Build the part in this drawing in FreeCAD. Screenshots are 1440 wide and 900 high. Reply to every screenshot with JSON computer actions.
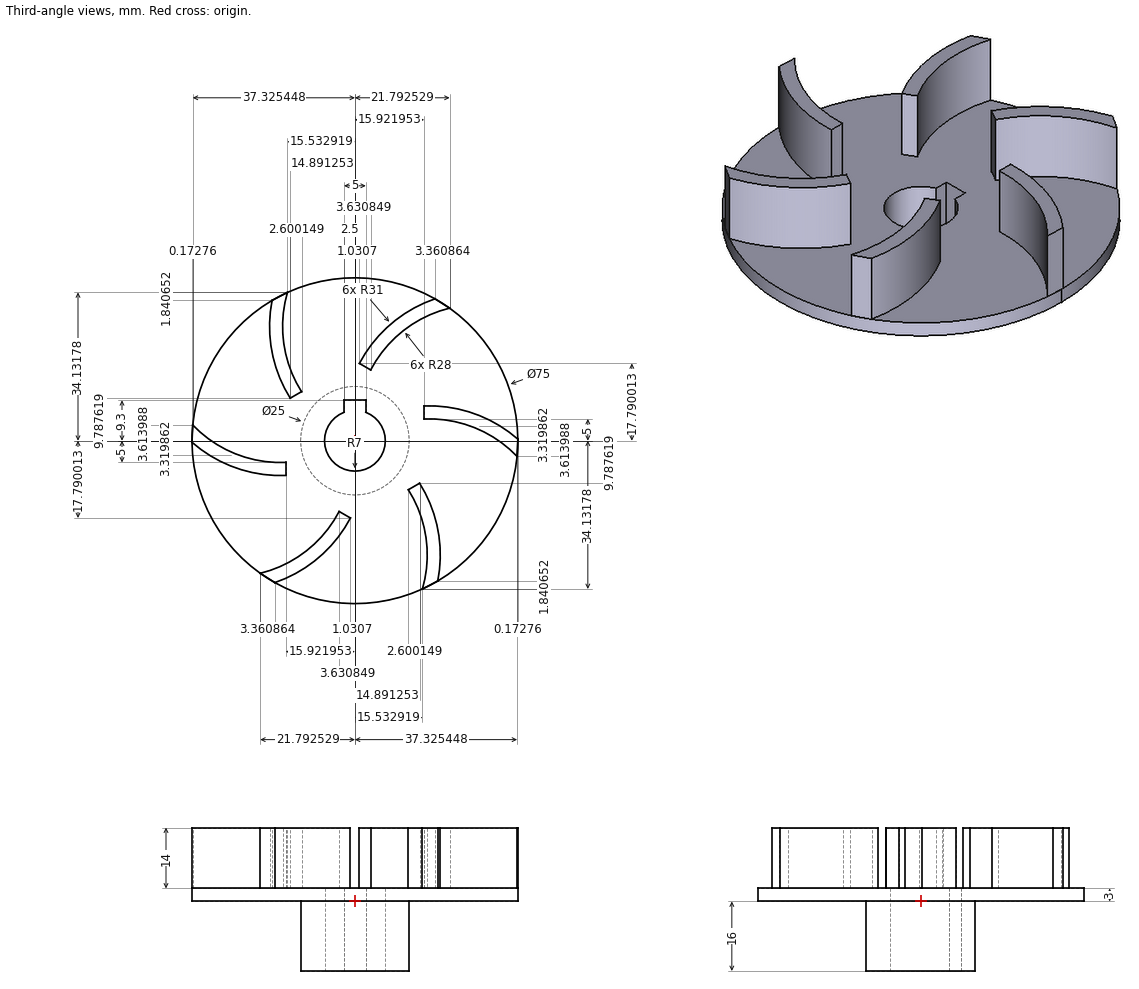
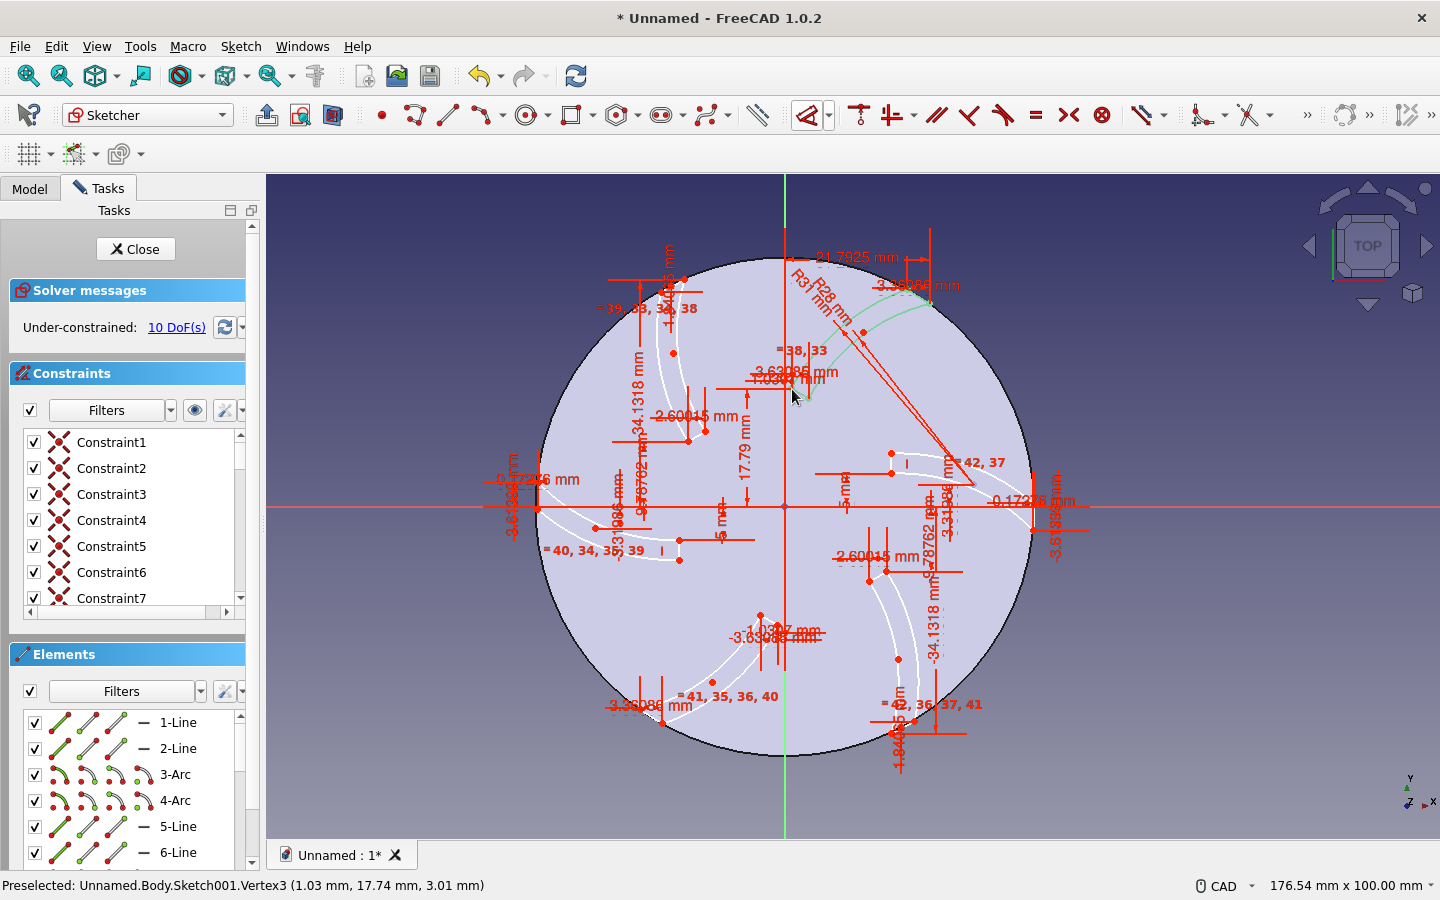
{"action": "left_click", "coordinate": [685, 280]}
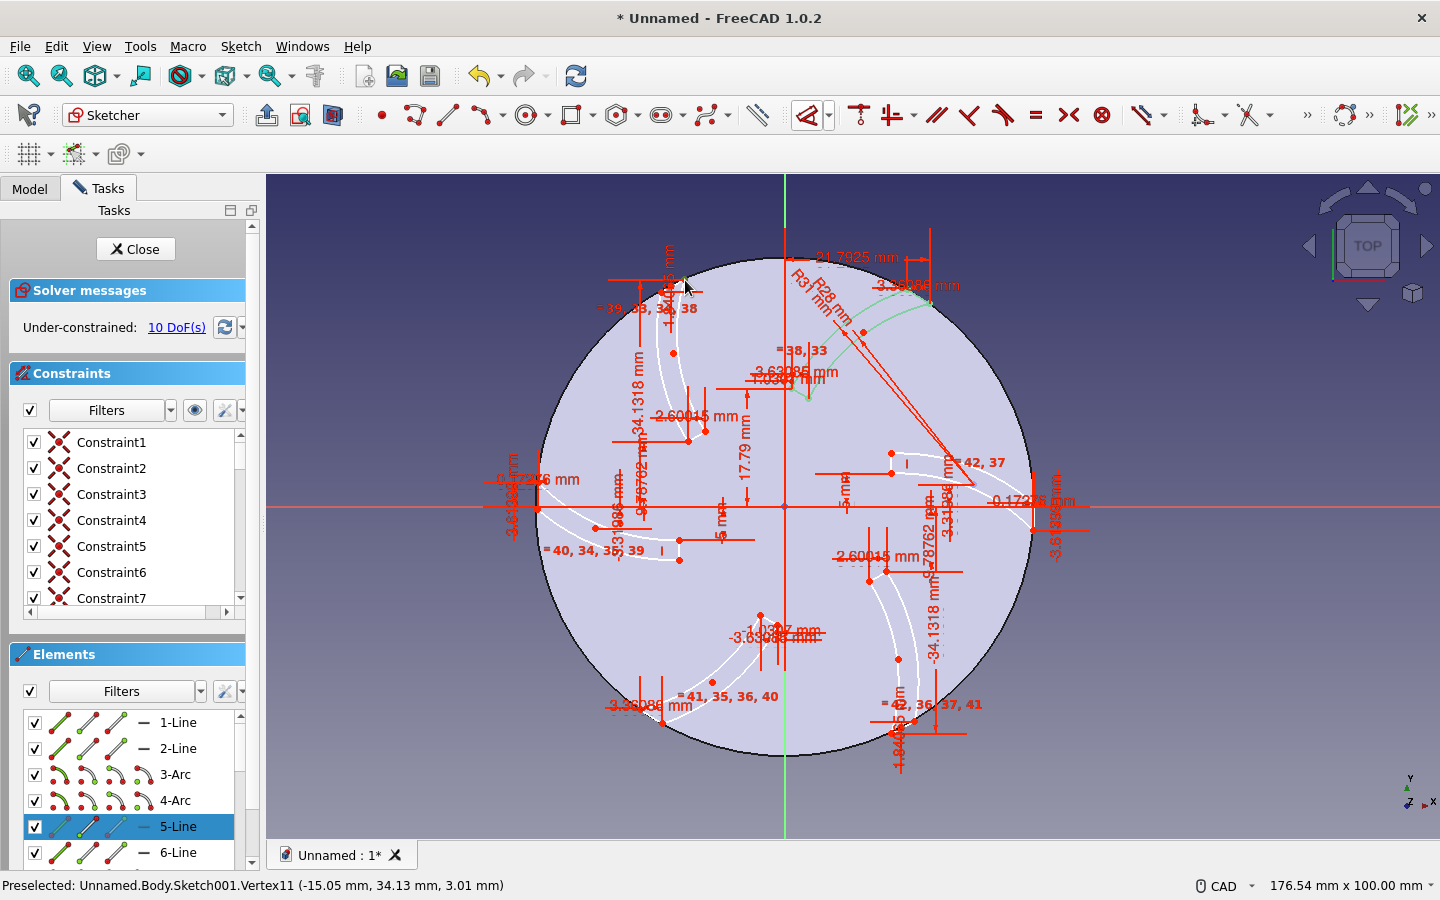
{"action": "left_click", "coordinate": [828, 116]}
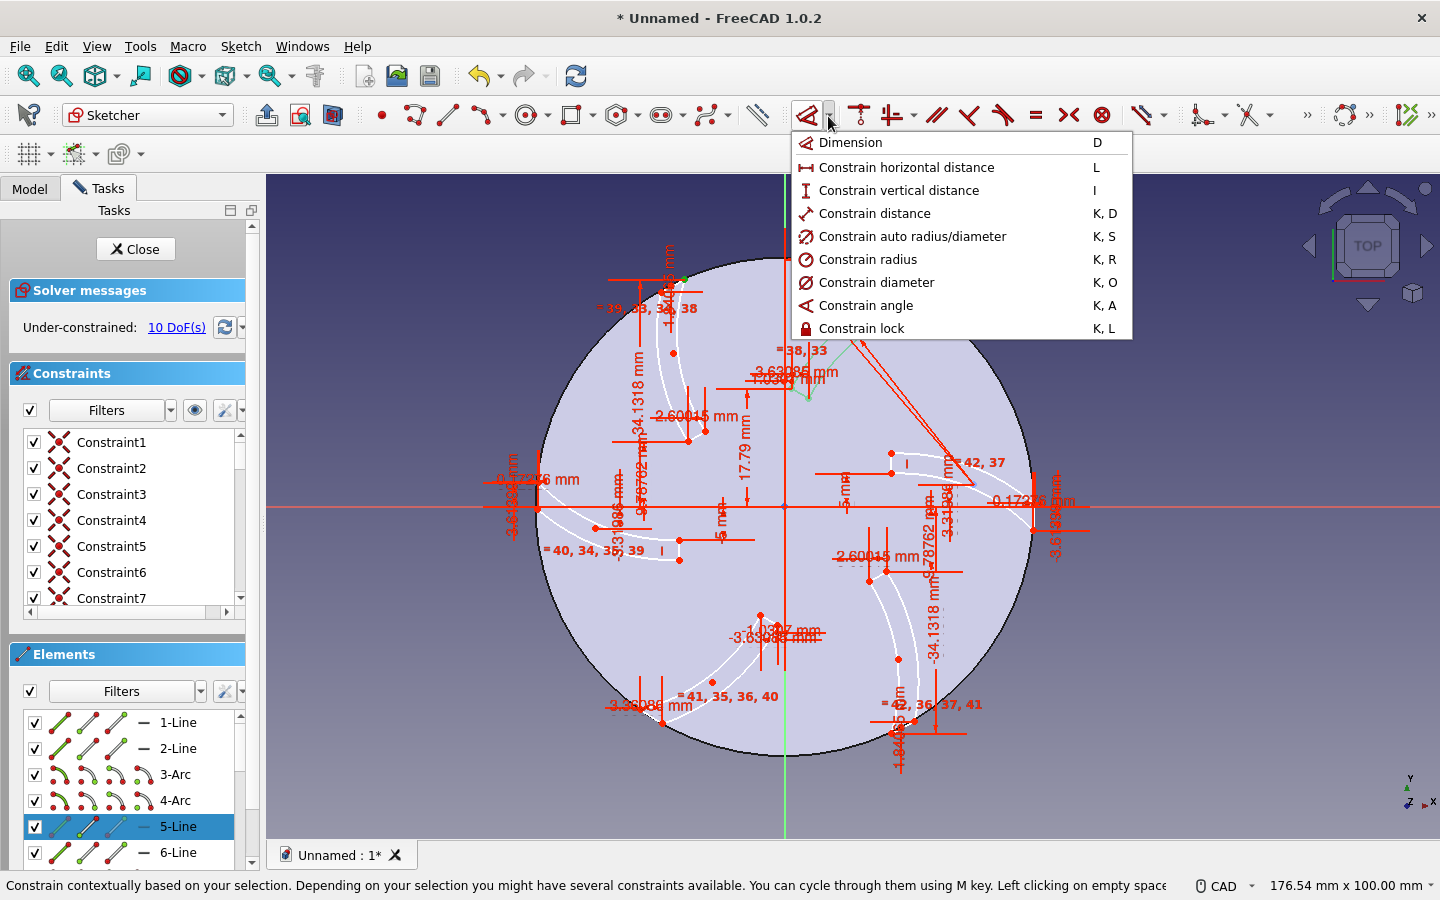
{"action": "left_click", "coordinate": [962, 168]}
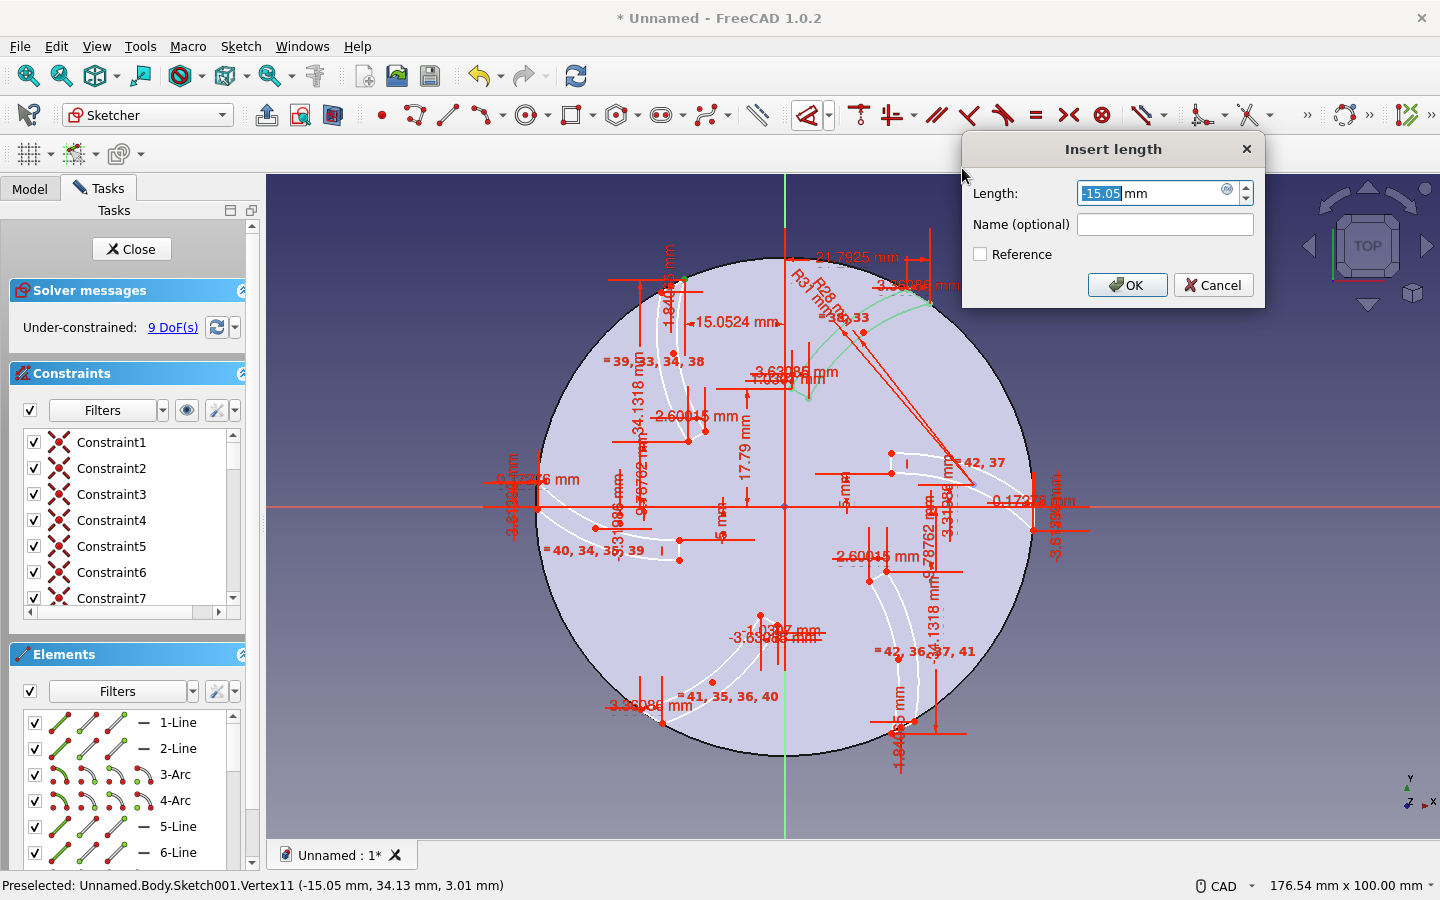
{"action": "type", "text": "-15.532919"}
{"action": "key", "text": "Return"}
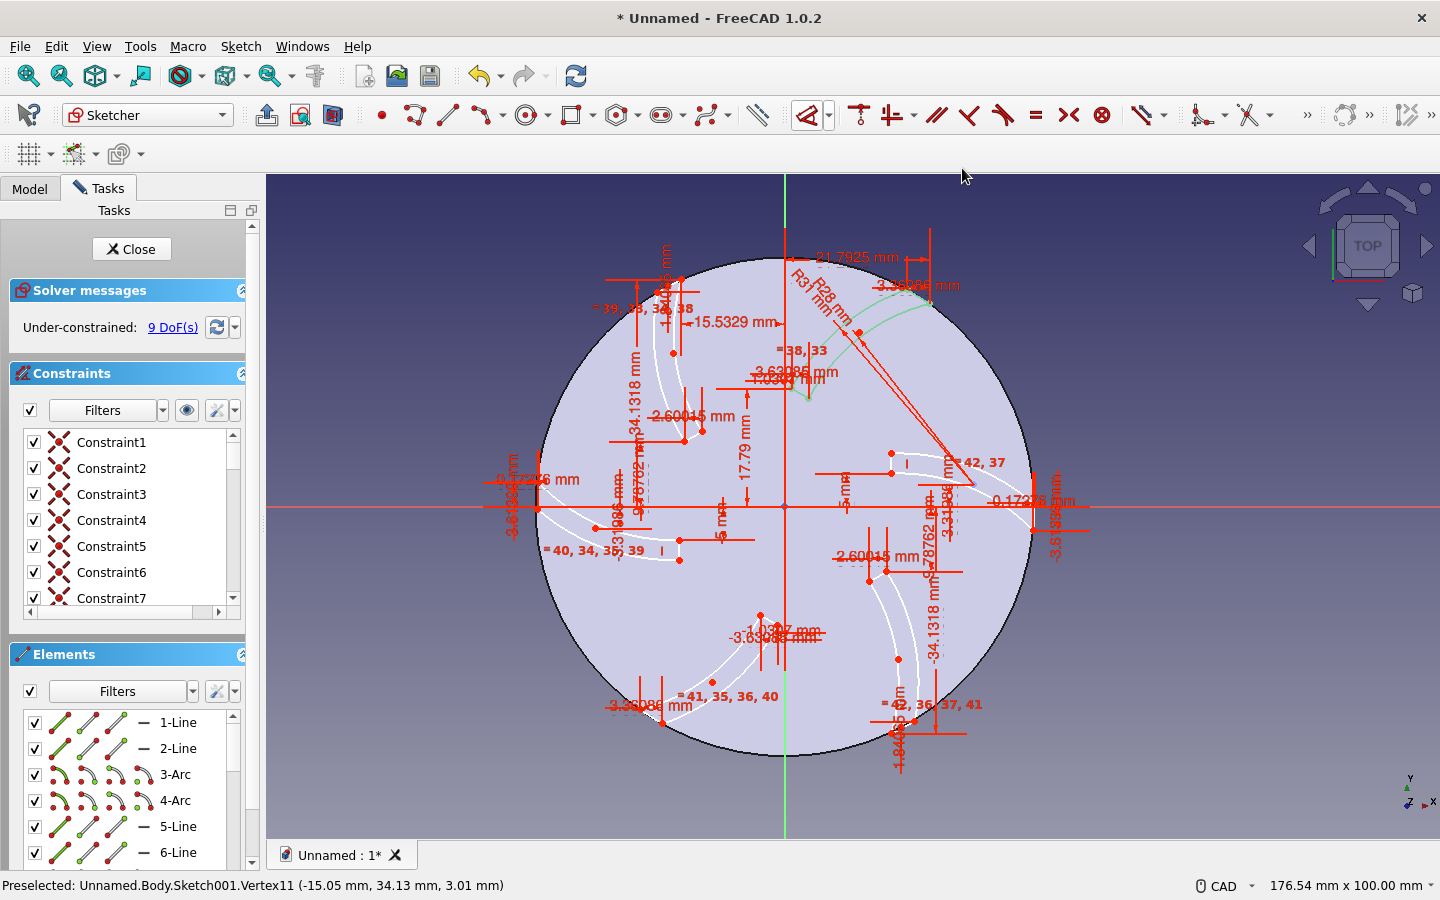
{"action": "left_click", "coordinate": [685, 442]}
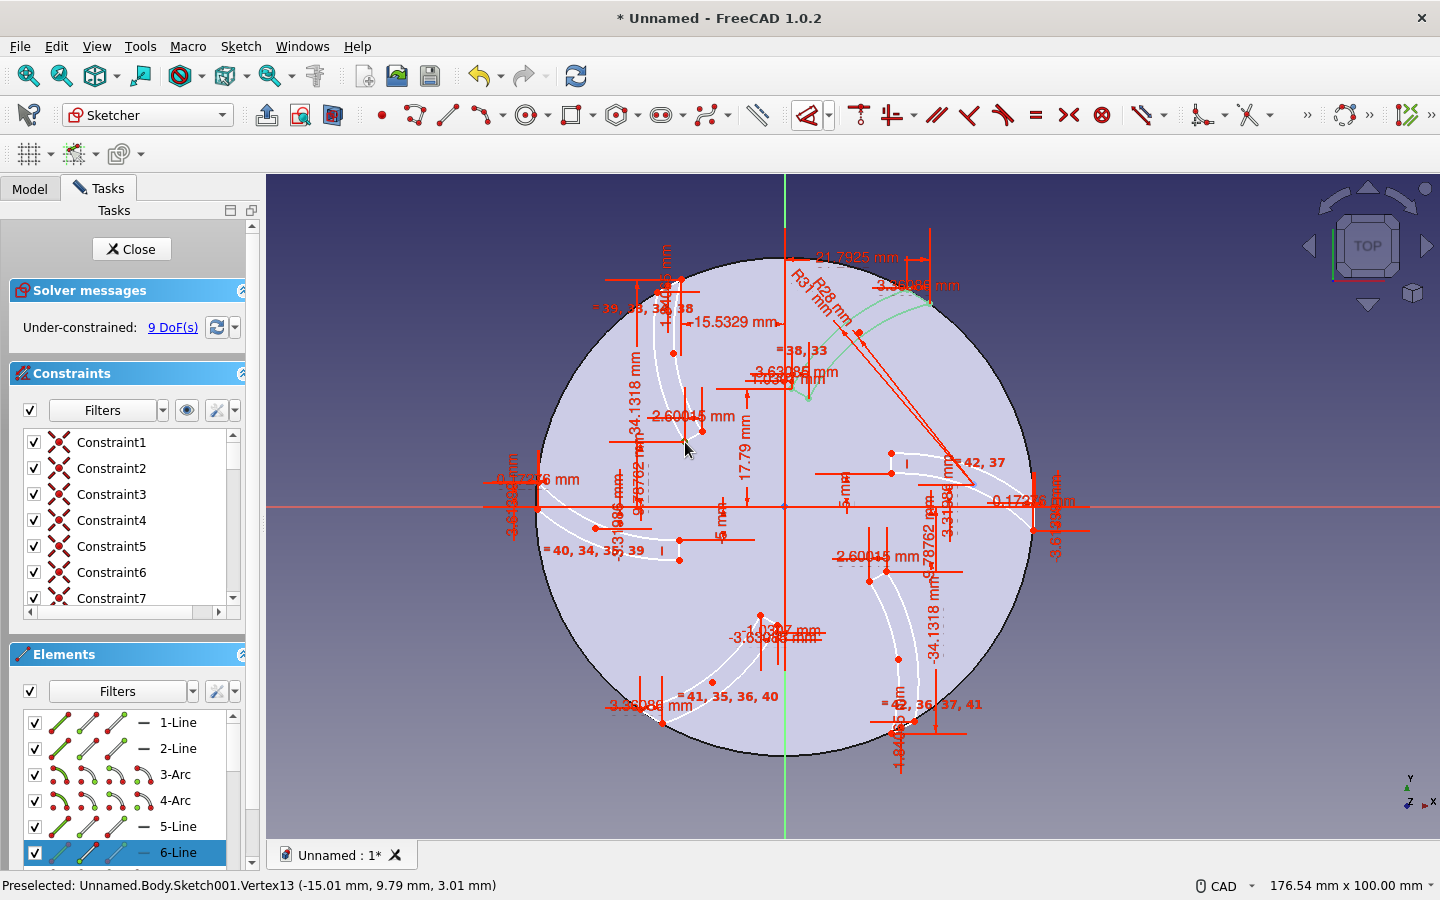
{"action": "key", "text": "l"}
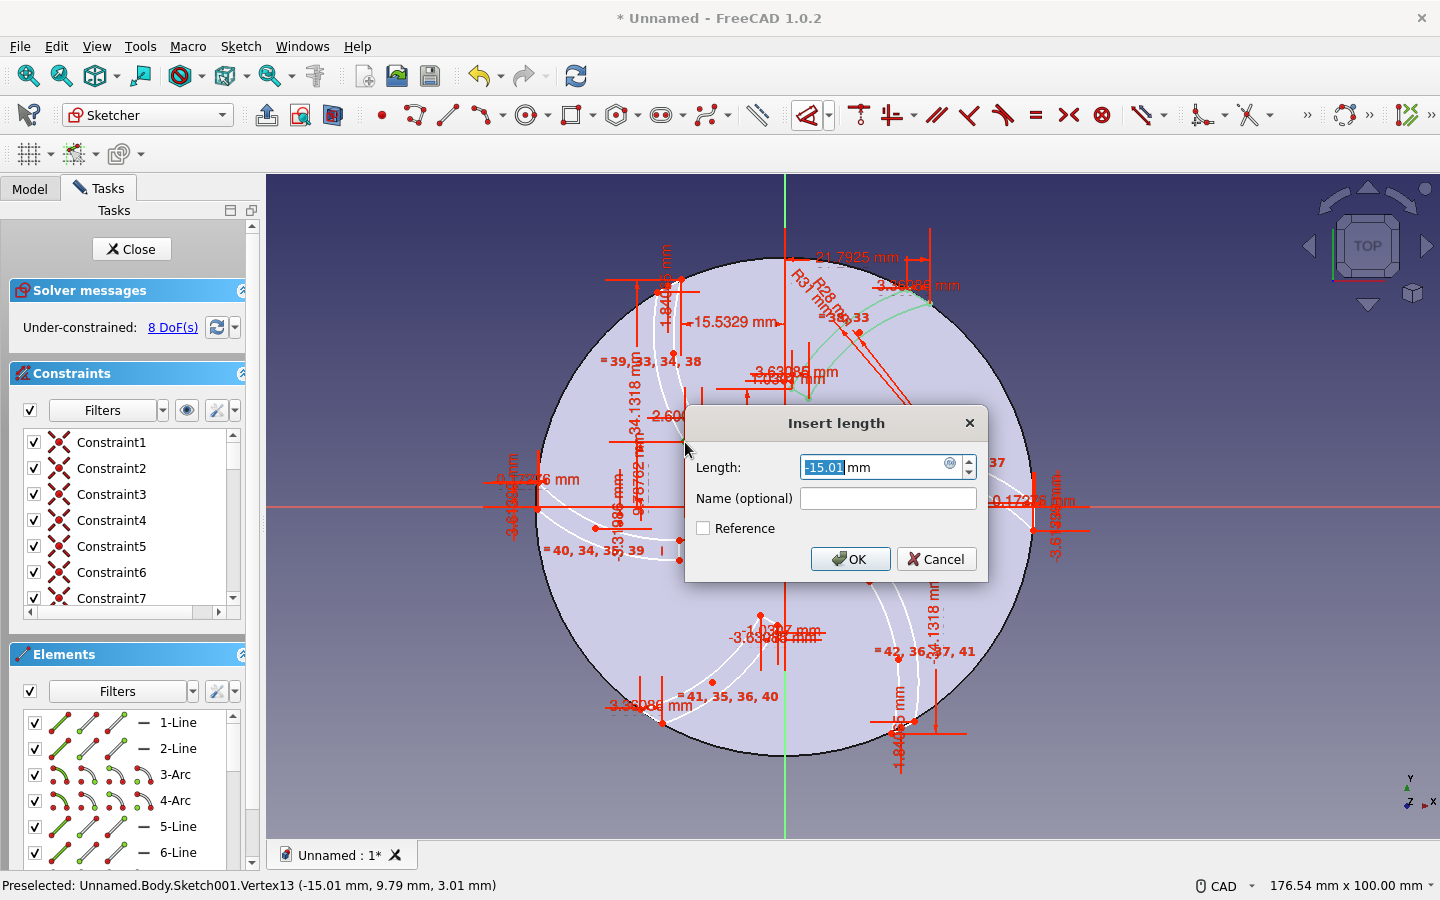
{"action": "type", "text": "-14.891253"}
{"action": "key", "text": "Return"}